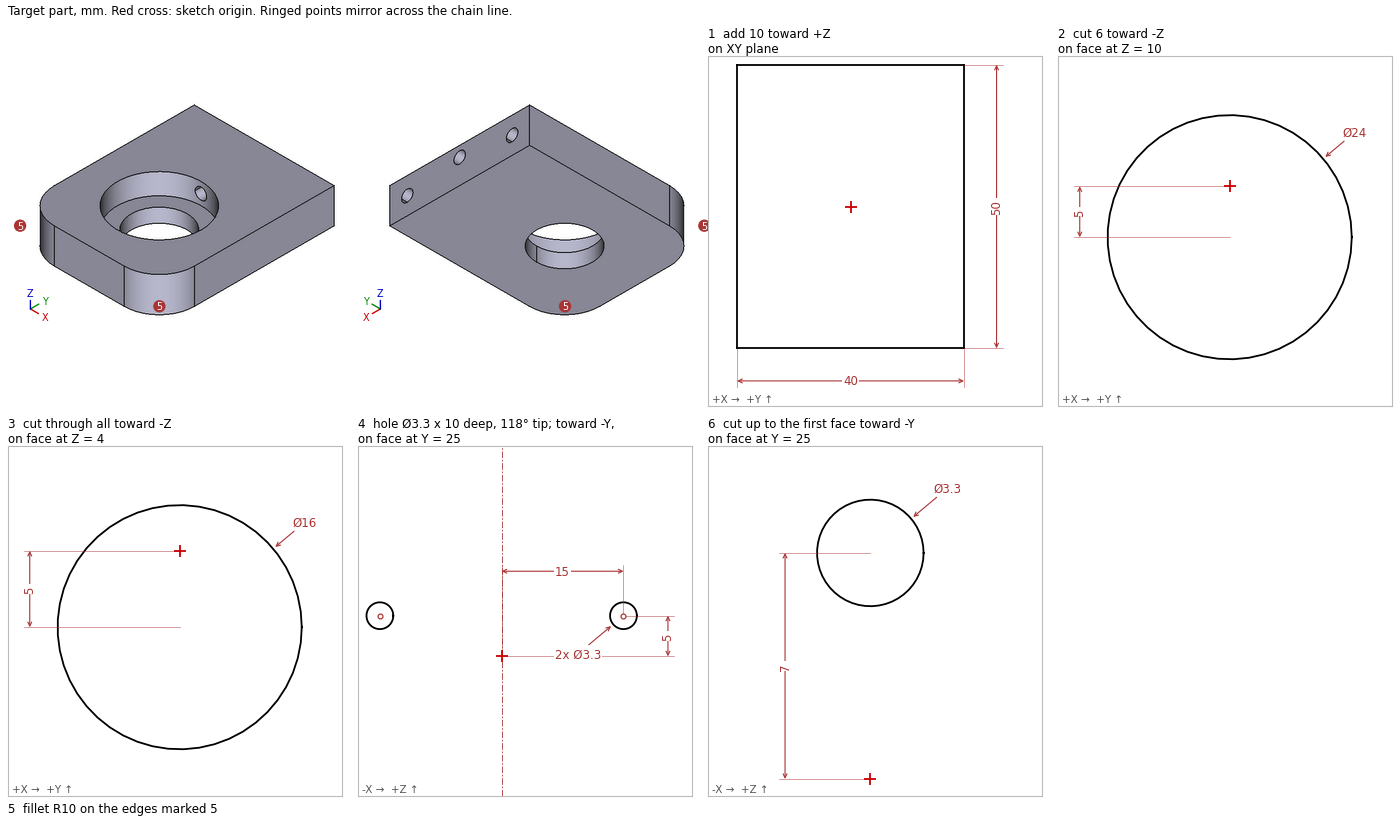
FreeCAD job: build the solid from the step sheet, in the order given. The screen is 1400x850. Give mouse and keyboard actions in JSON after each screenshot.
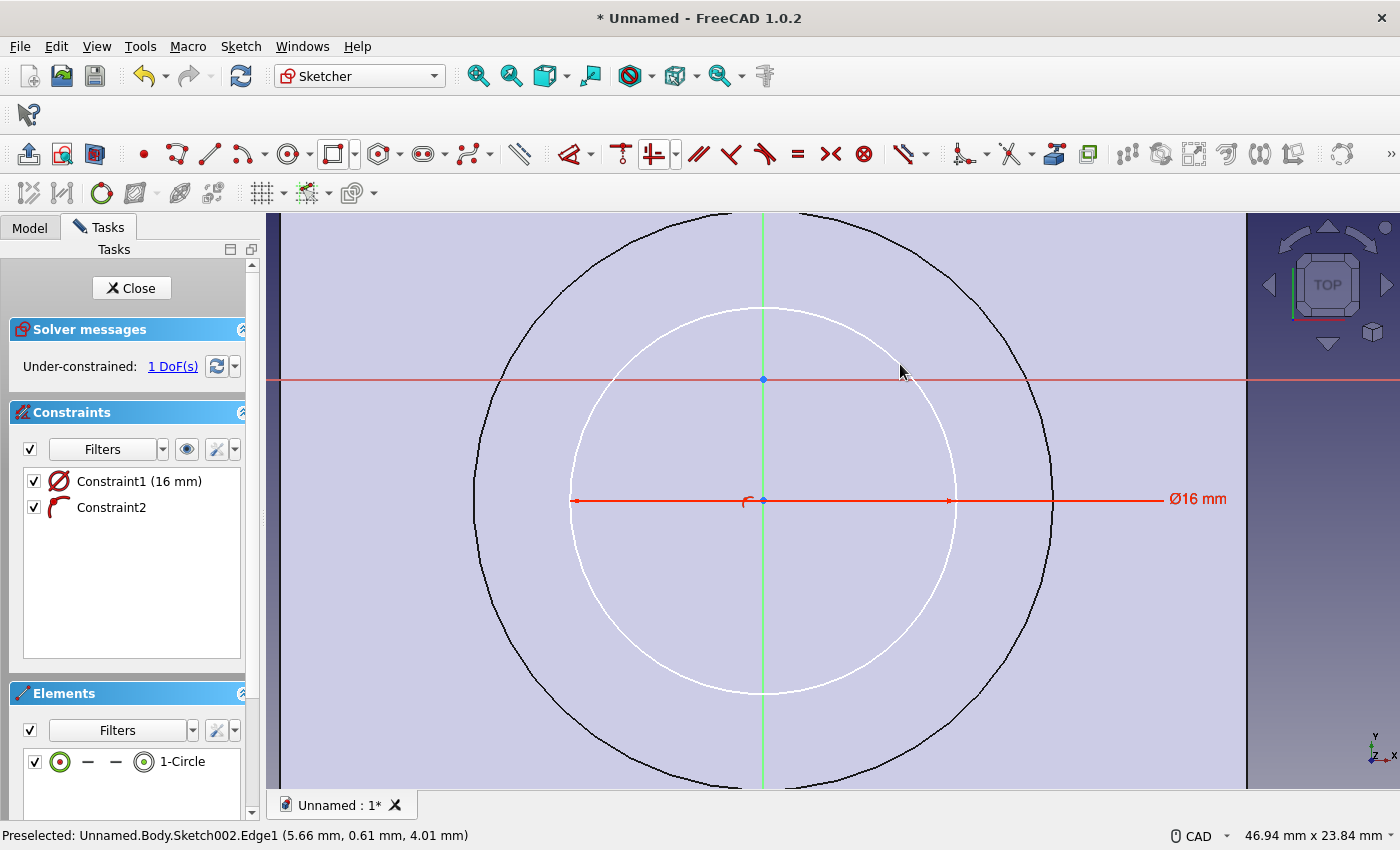
{"action": "left_click", "coordinate": [568, 154]}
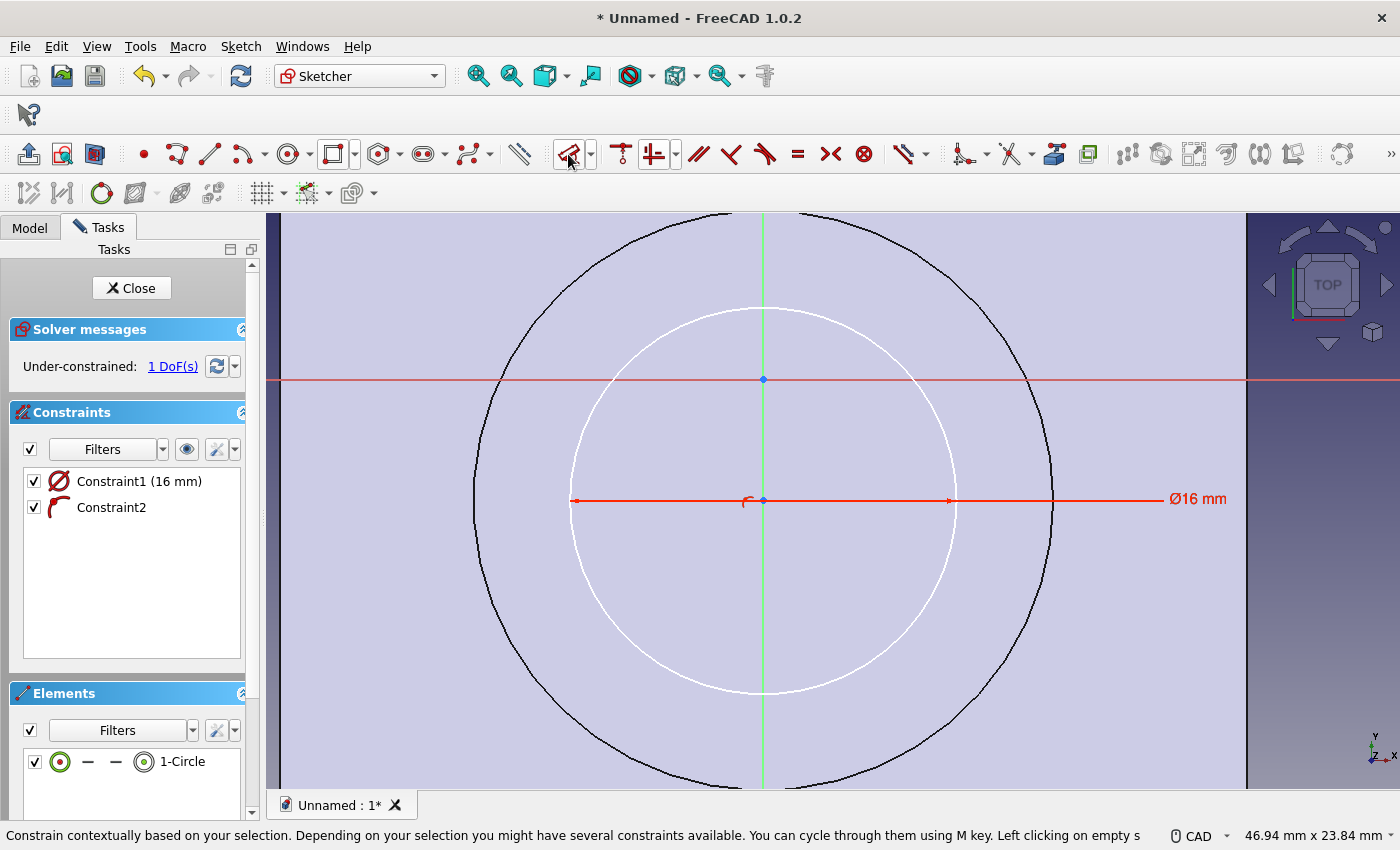
{"action": "left_click", "coordinate": [763, 501]}
{"action": "left_click", "coordinate": [797, 440]}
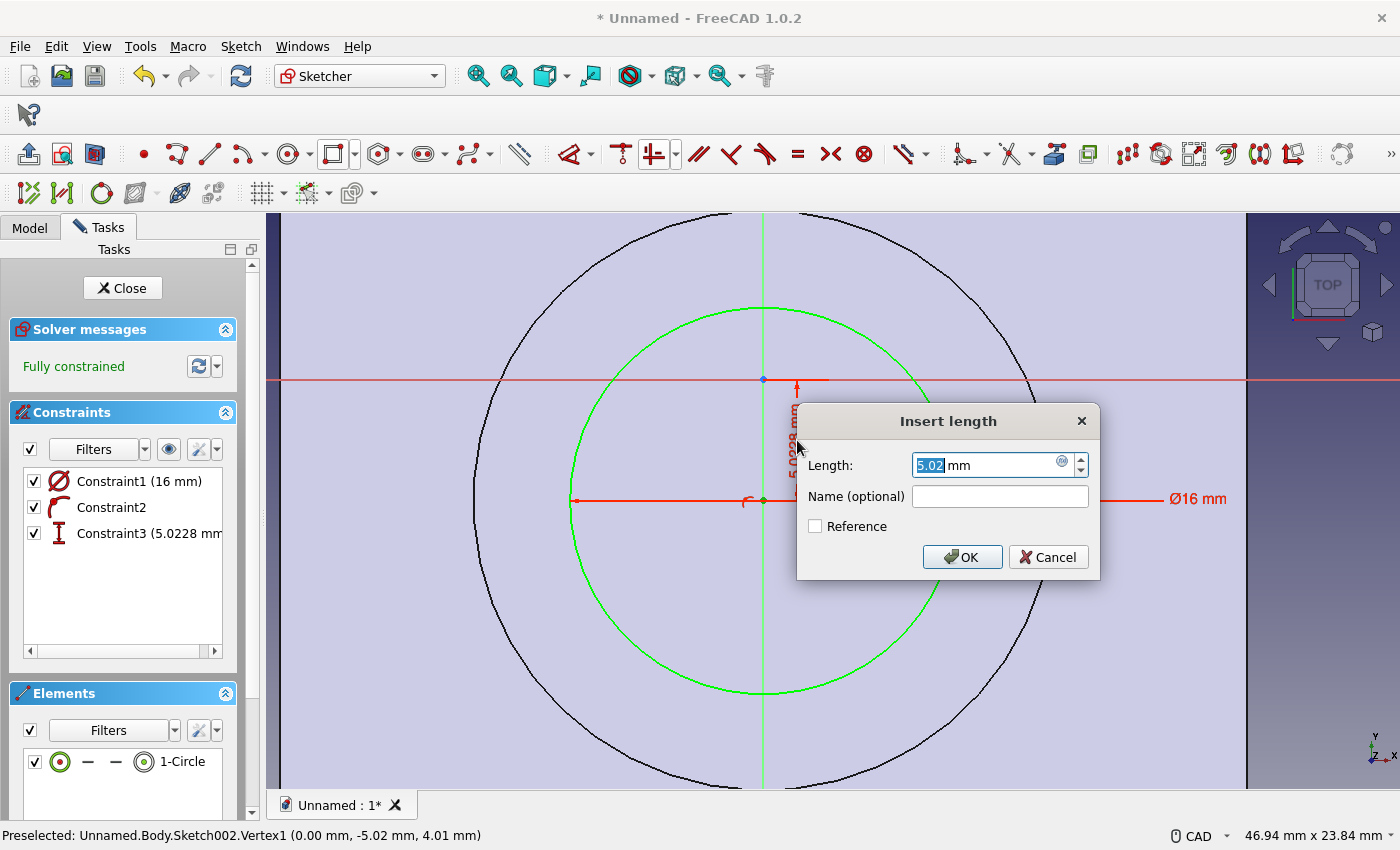
{"action": "type", "text": "5"}
{"action": "key", "text": "Return"}
{"action": "key", "text": "Escape"}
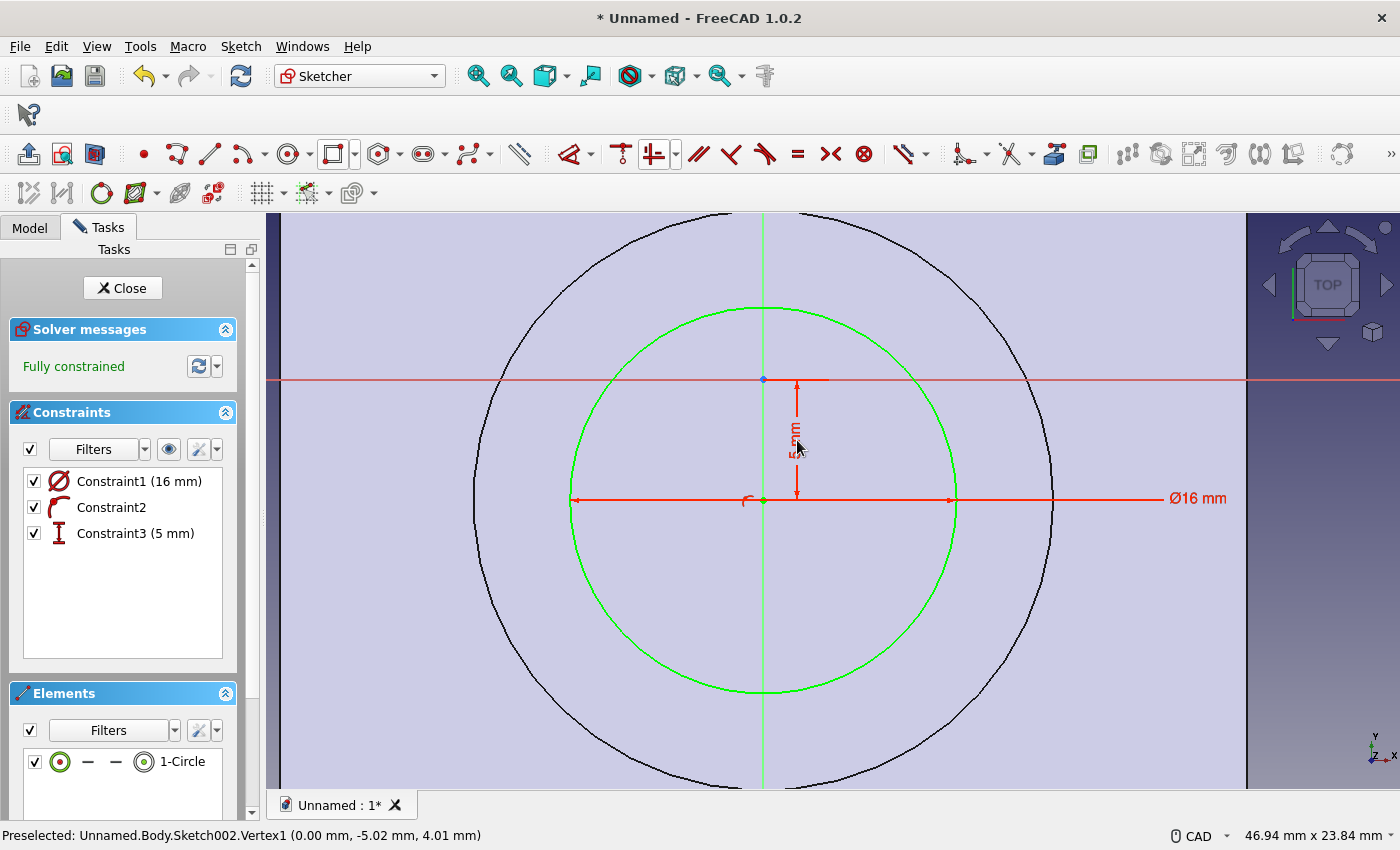
{"action": "left_click", "coordinate": [123, 288]}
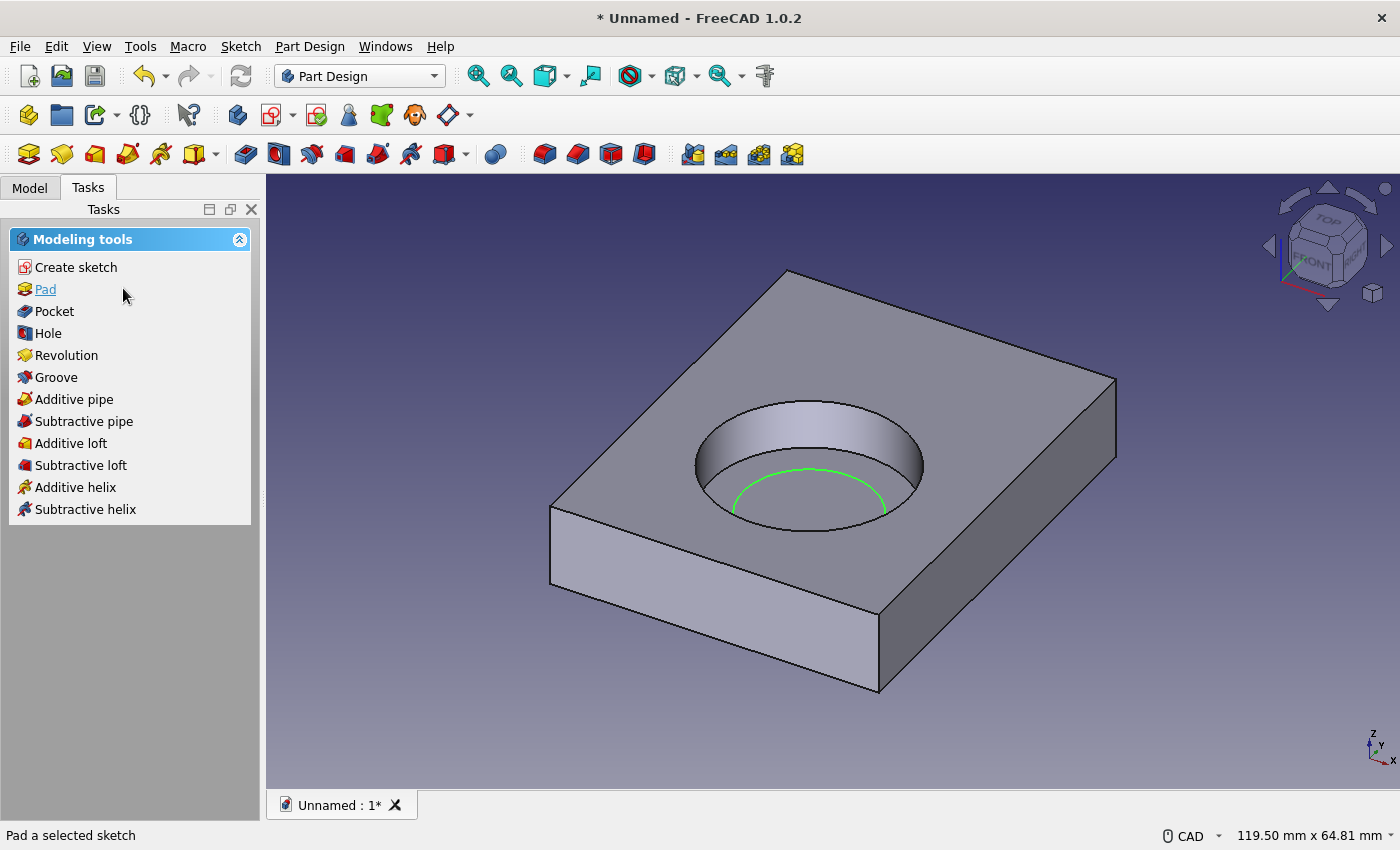
{"action": "left_click", "coordinate": [246, 154]}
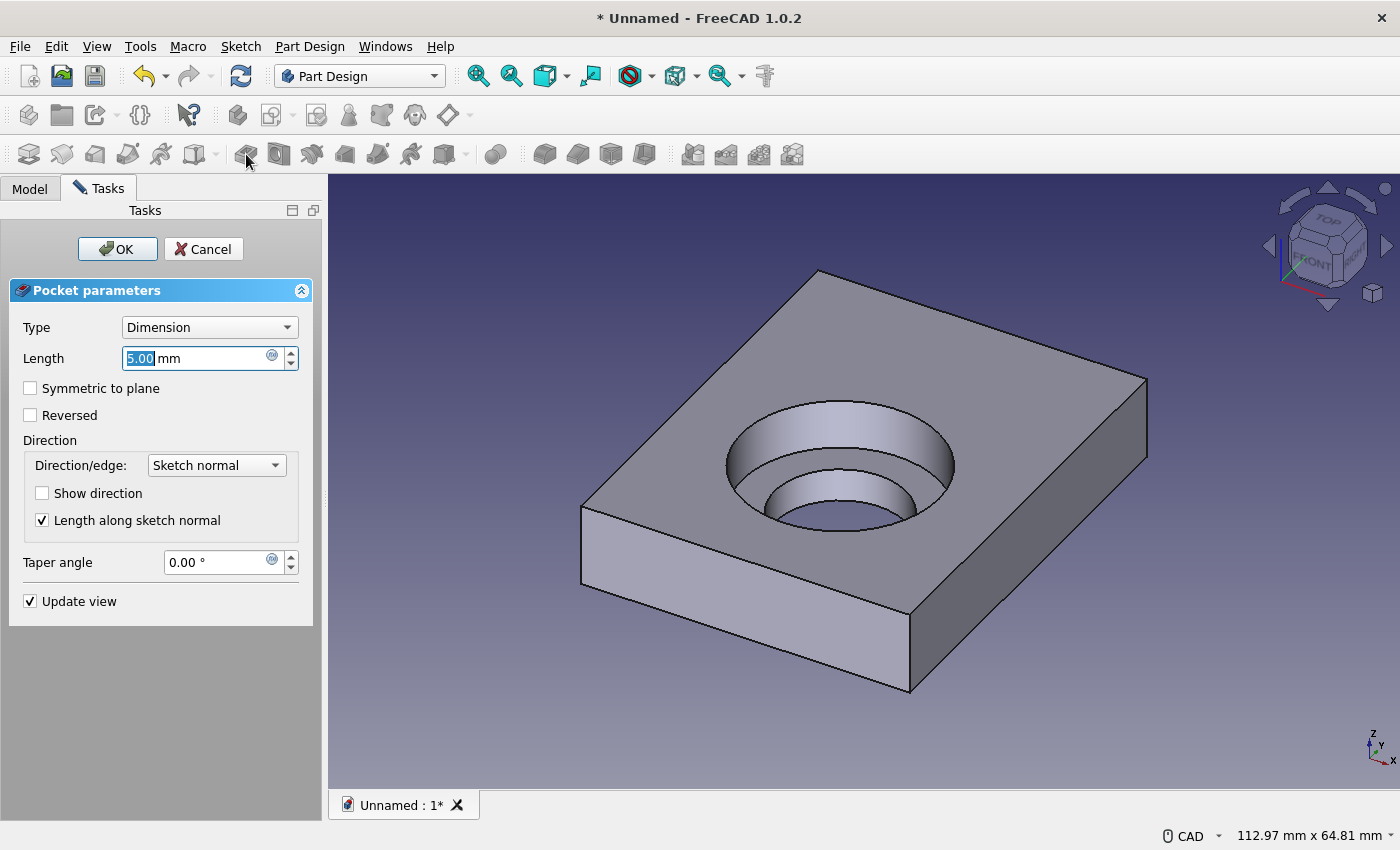
{"action": "left_click", "coordinate": [210, 328]}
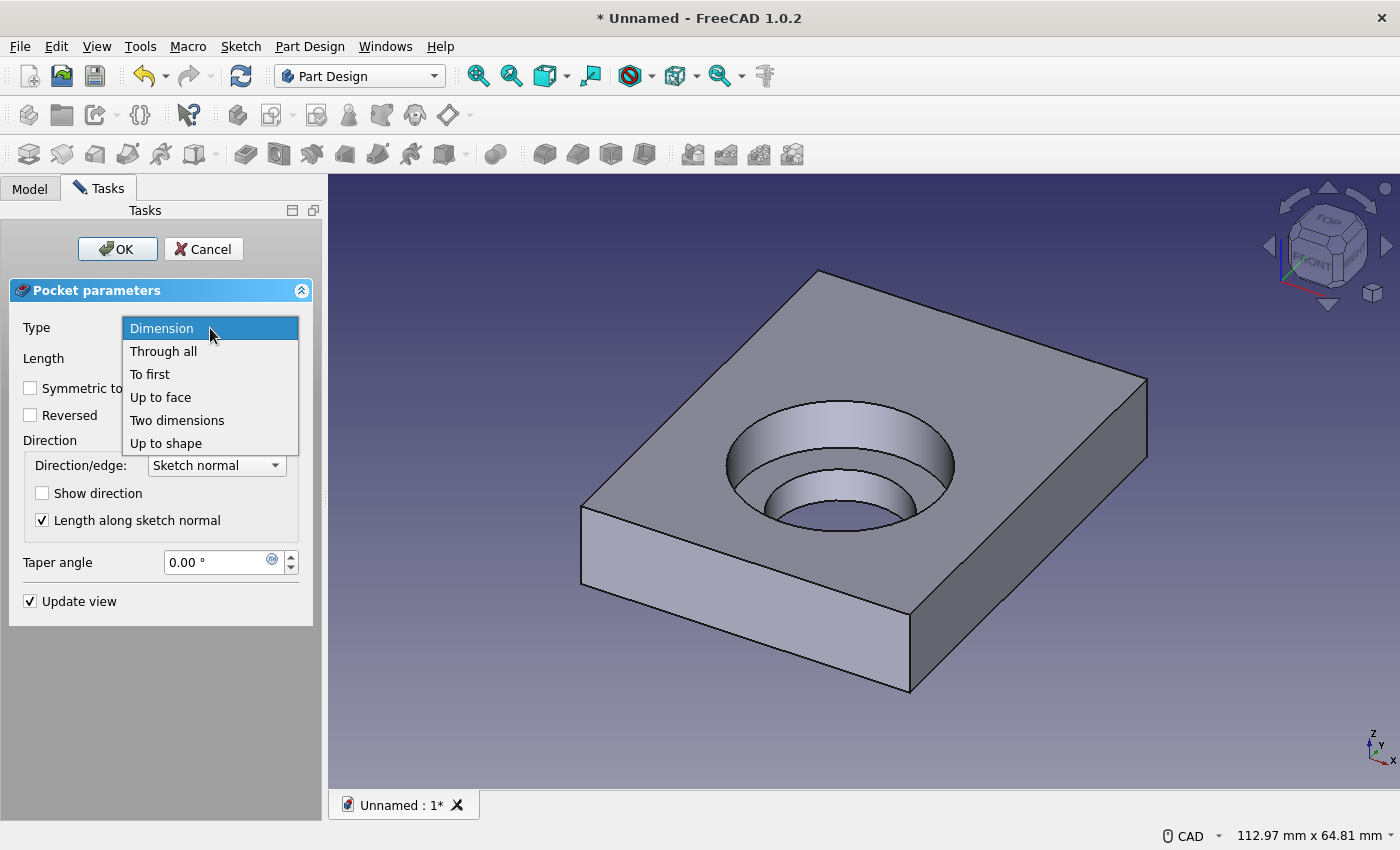
{"action": "left_click", "coordinate": [208, 352]}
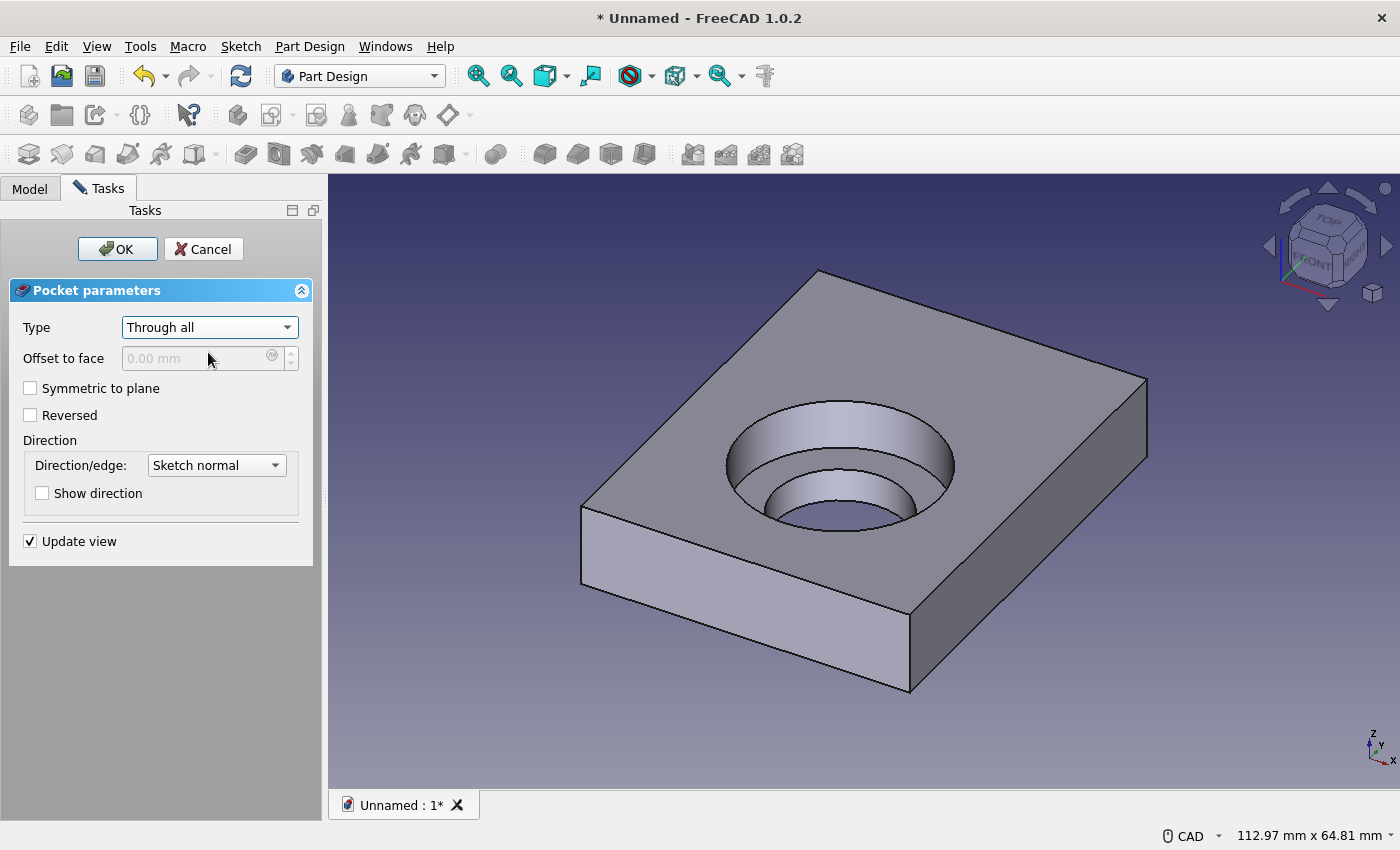
{"action": "left_click", "coordinate": [118, 249]}